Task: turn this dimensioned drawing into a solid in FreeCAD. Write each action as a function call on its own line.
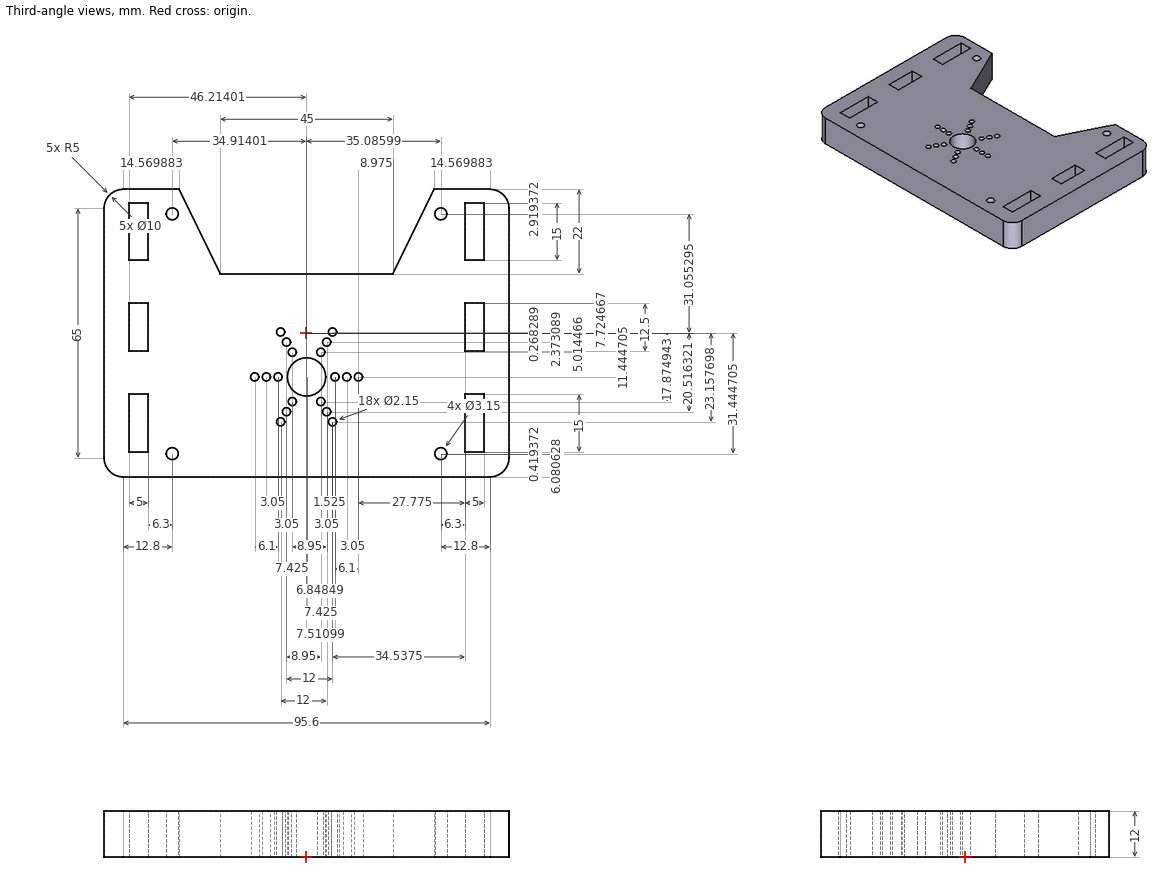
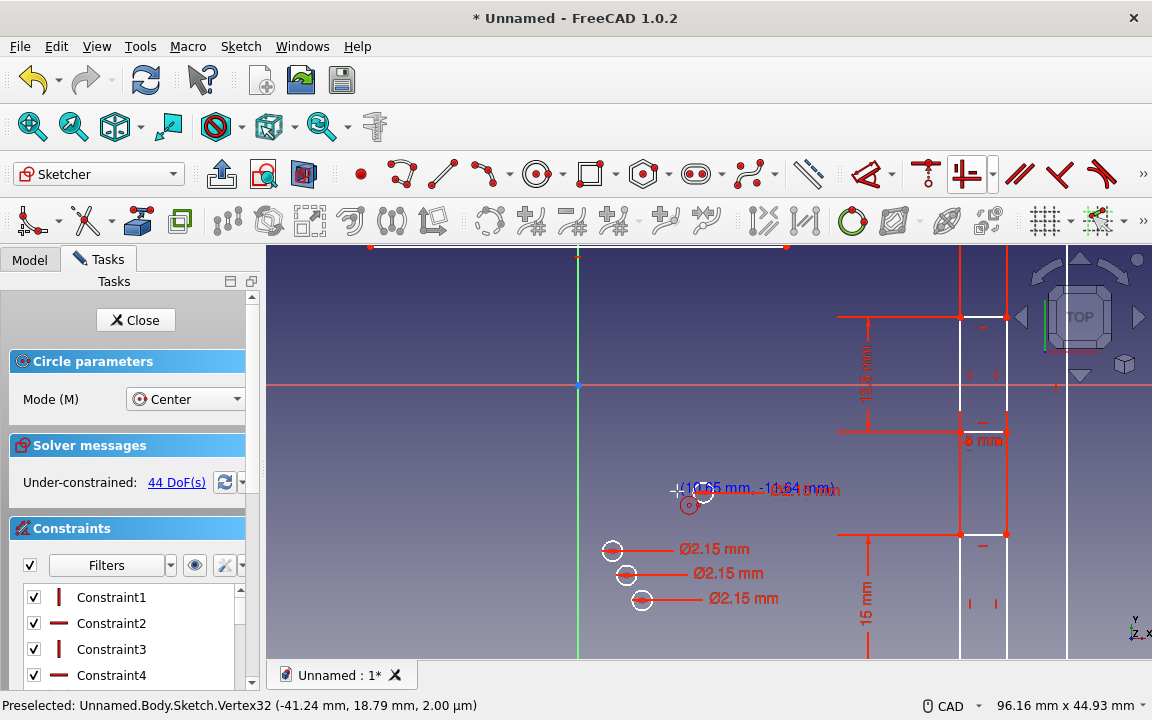
click(675, 491)
move(668, 484)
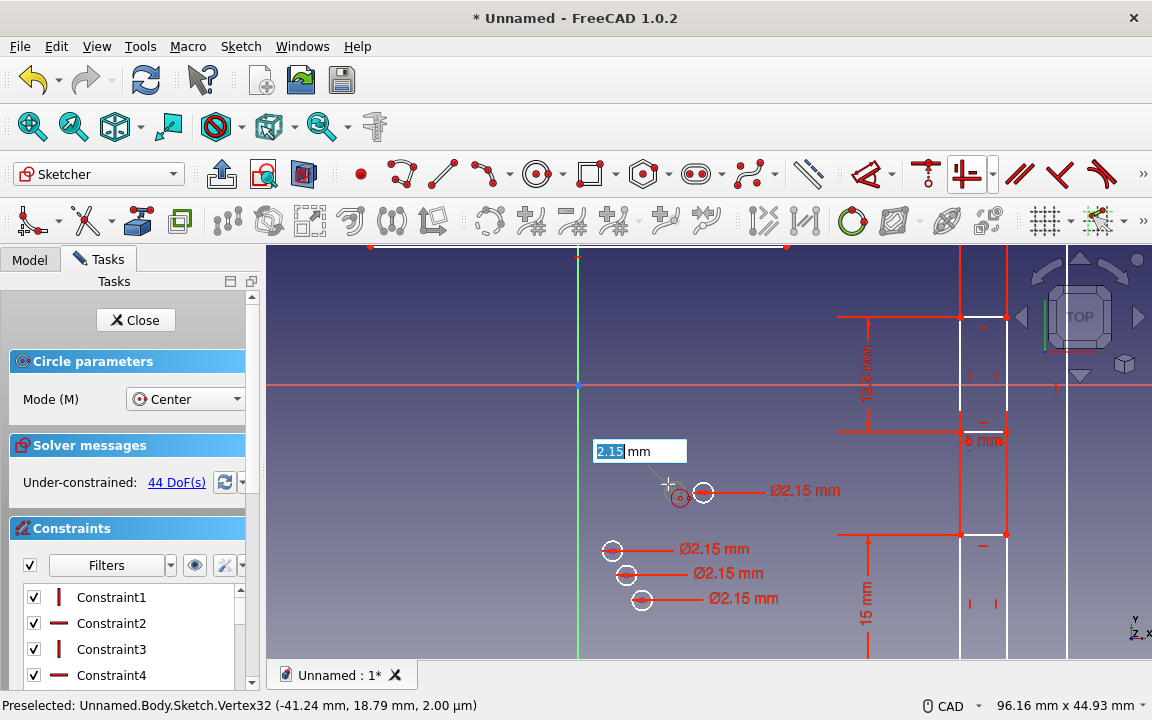
text(2.15)
key(Return)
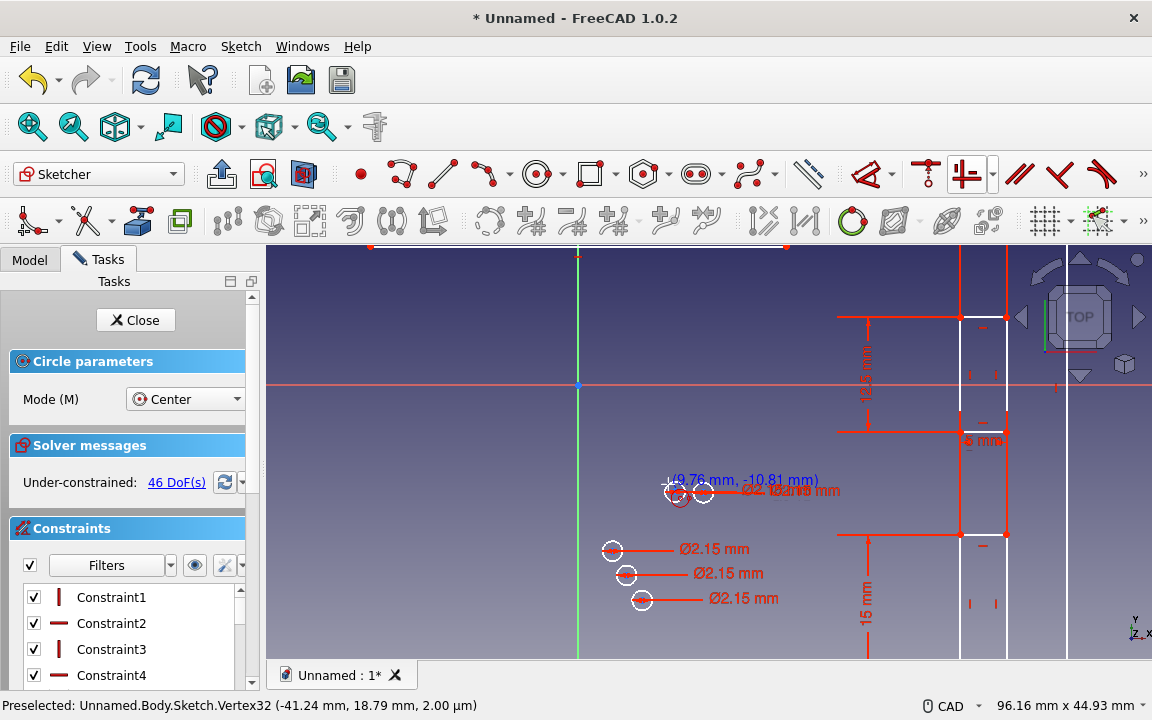
scroll(647, 491, up, 5)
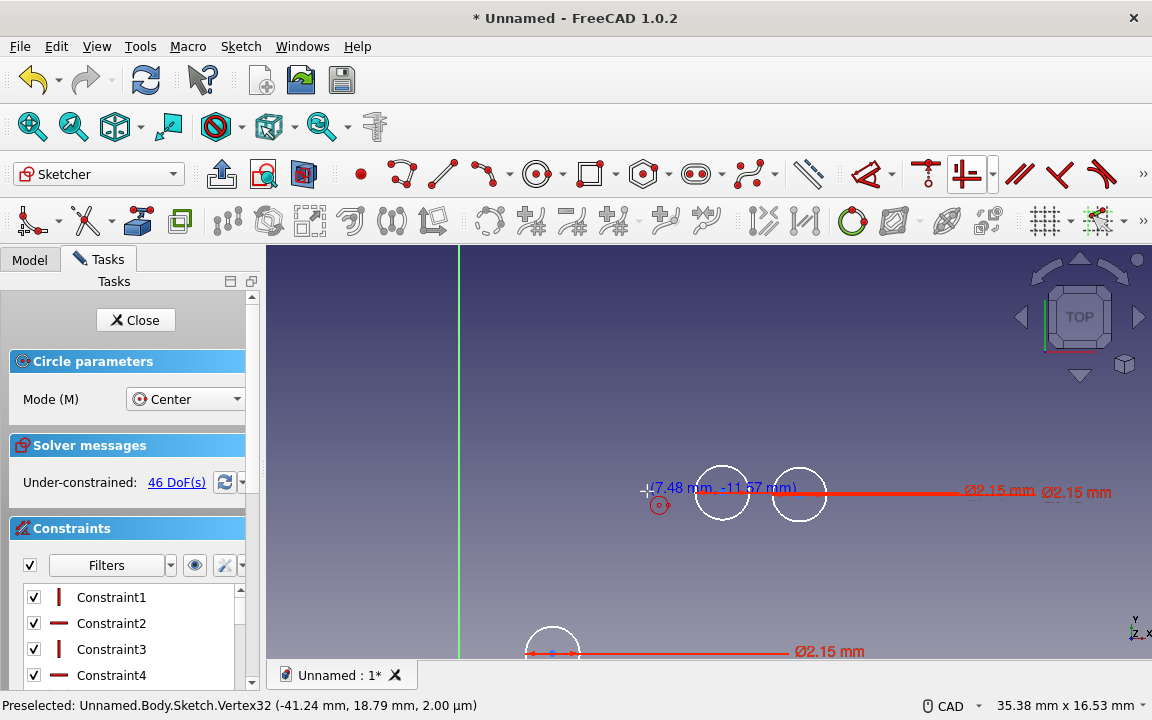
scroll(669, 491, down, 10)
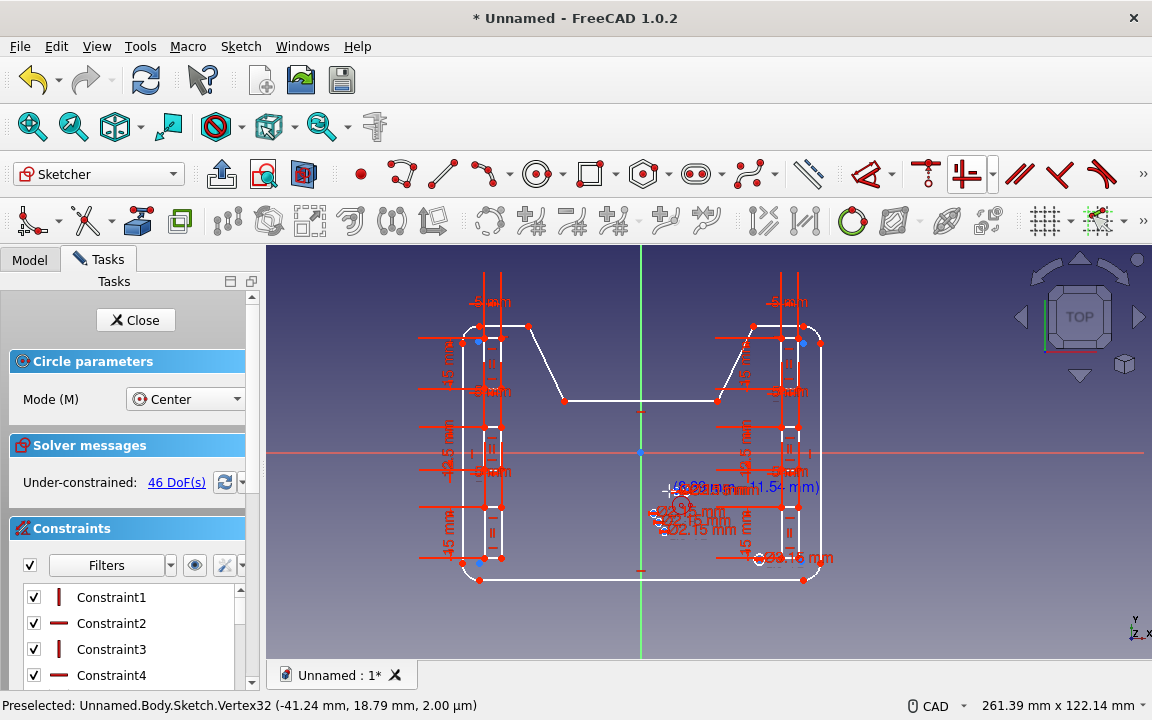
scroll(666, 491, up, 5)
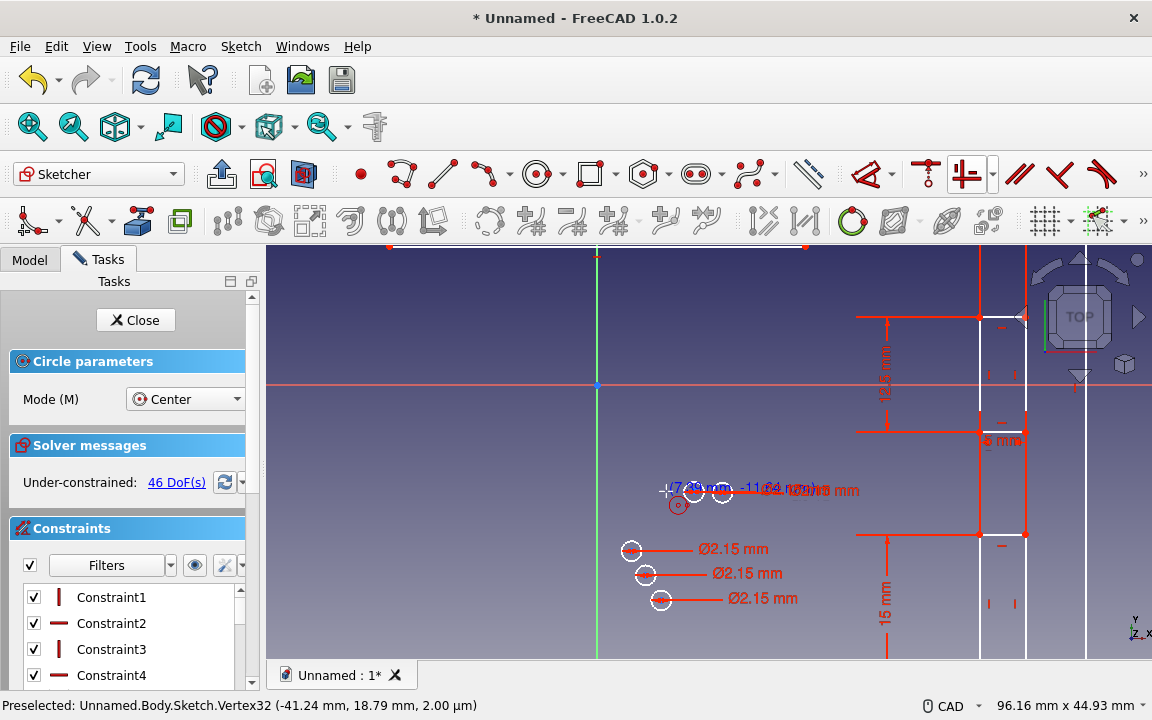
click(666, 491)
move(659, 484)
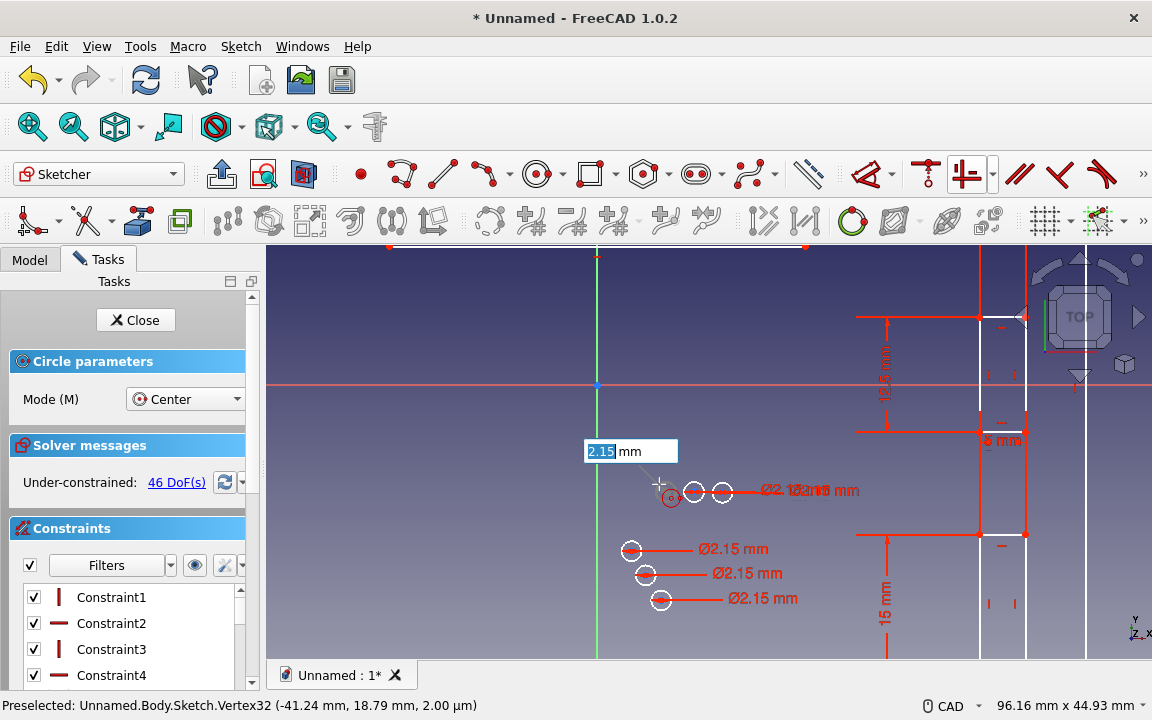
text(2.15)
key(Return)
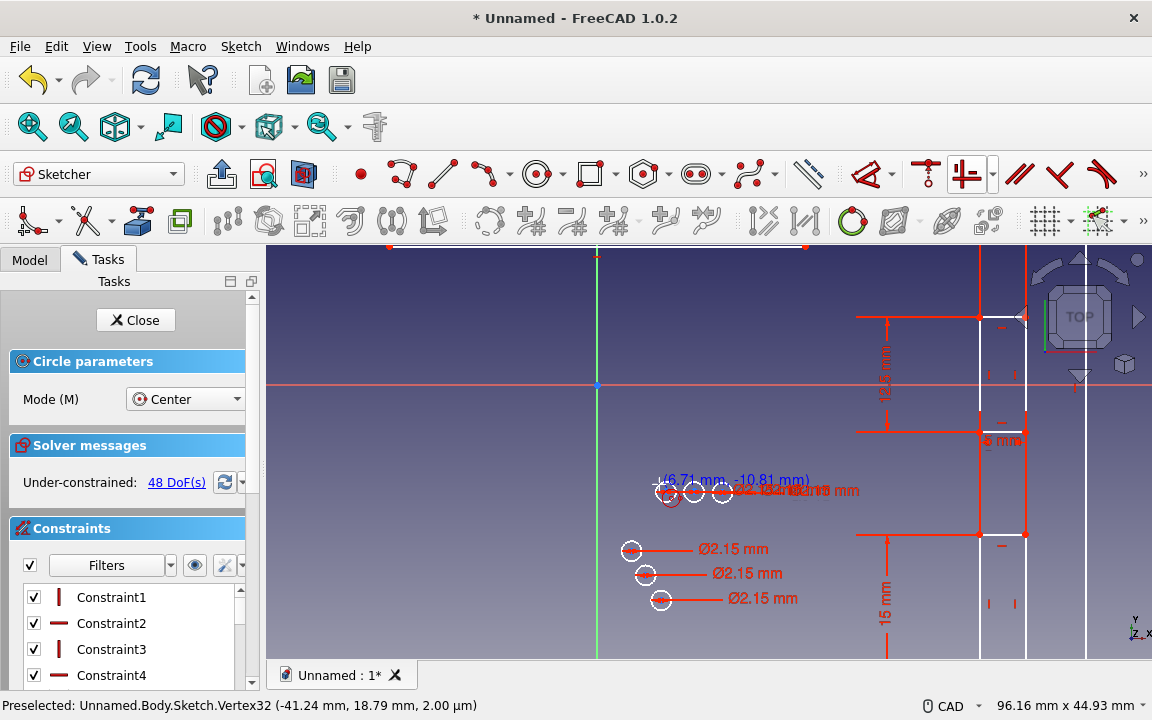
scroll(632, 432, up, 5)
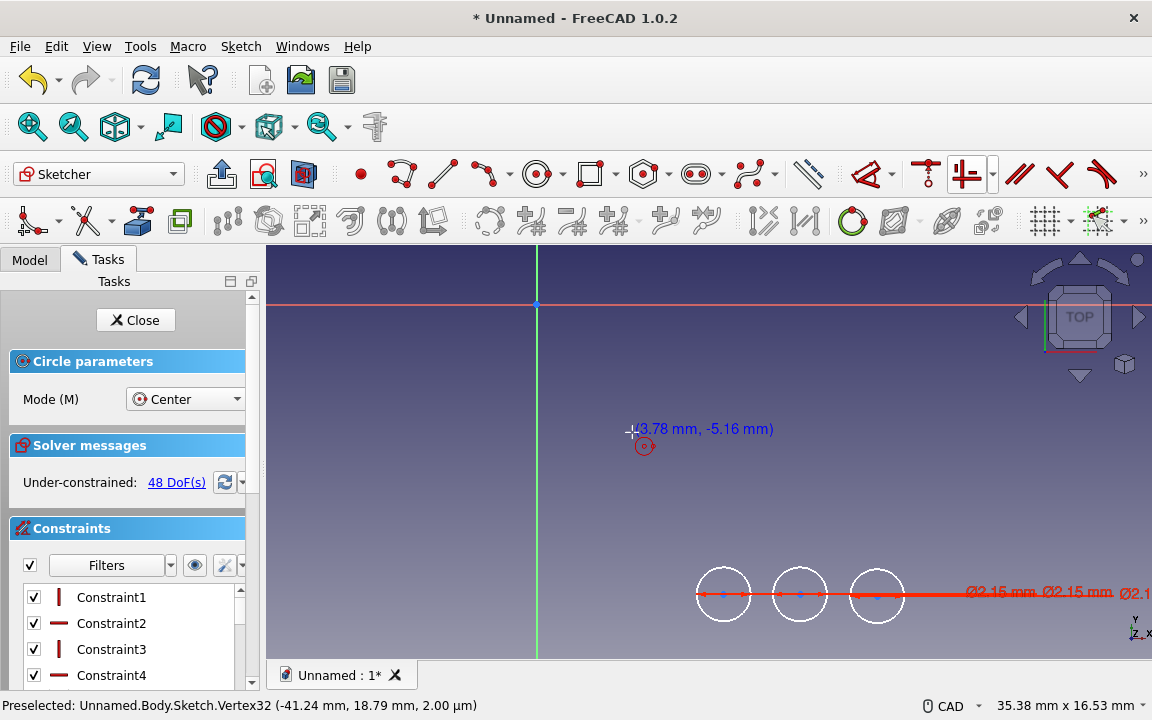
scroll(656, 475, down, 10)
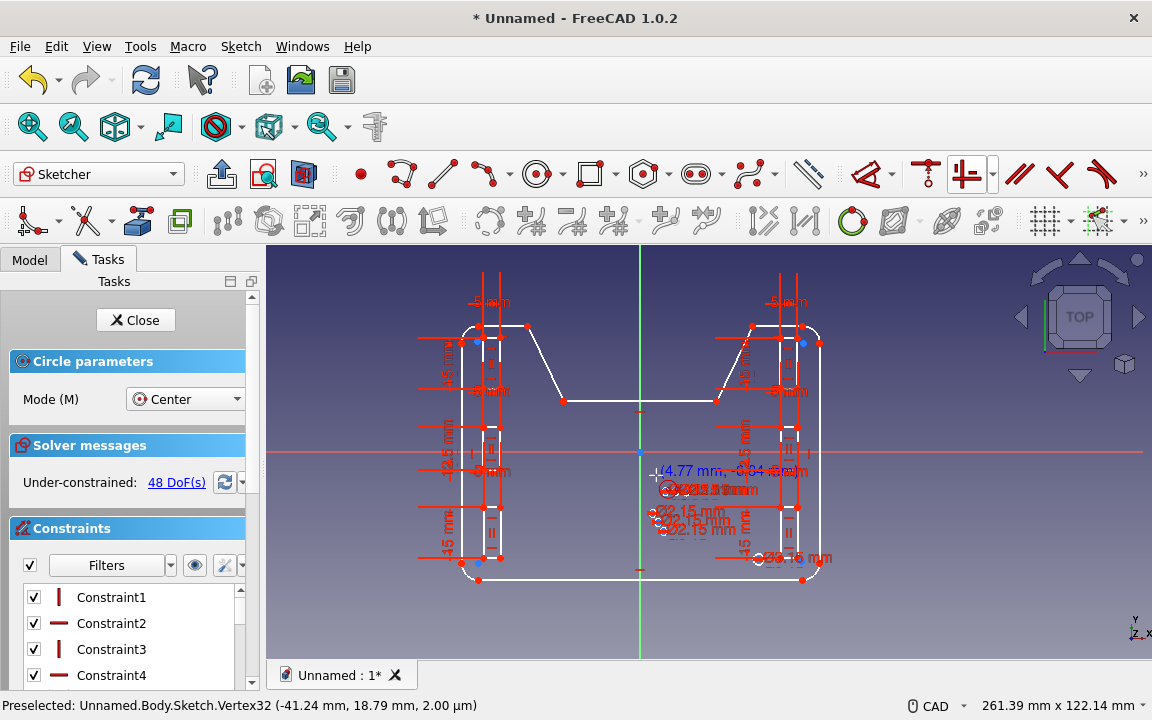
scroll(653, 469, up, 2)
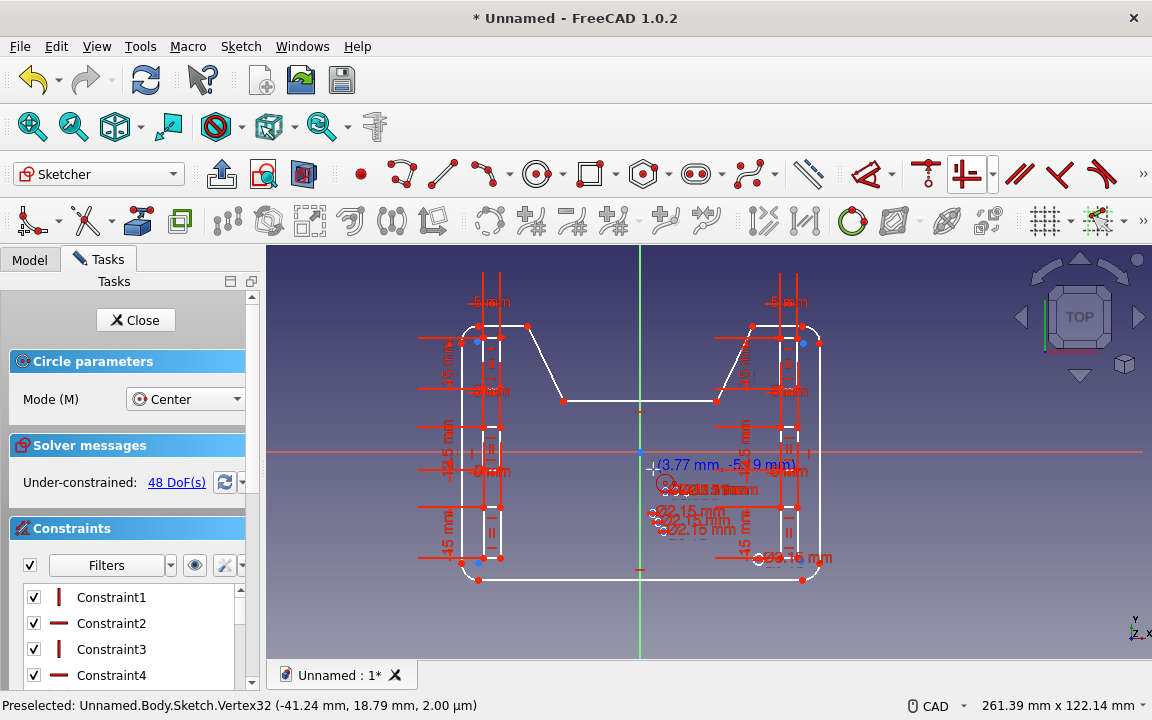
click(653, 469)
move(657, 466)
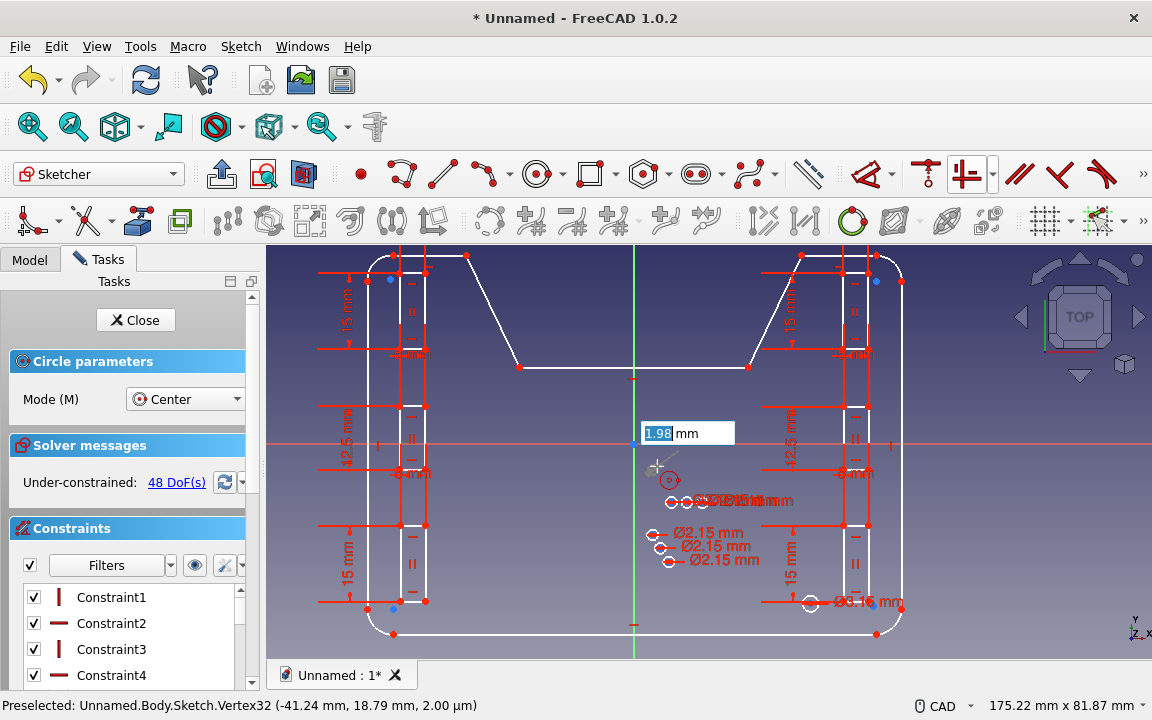
text(2.15)
key(Return)